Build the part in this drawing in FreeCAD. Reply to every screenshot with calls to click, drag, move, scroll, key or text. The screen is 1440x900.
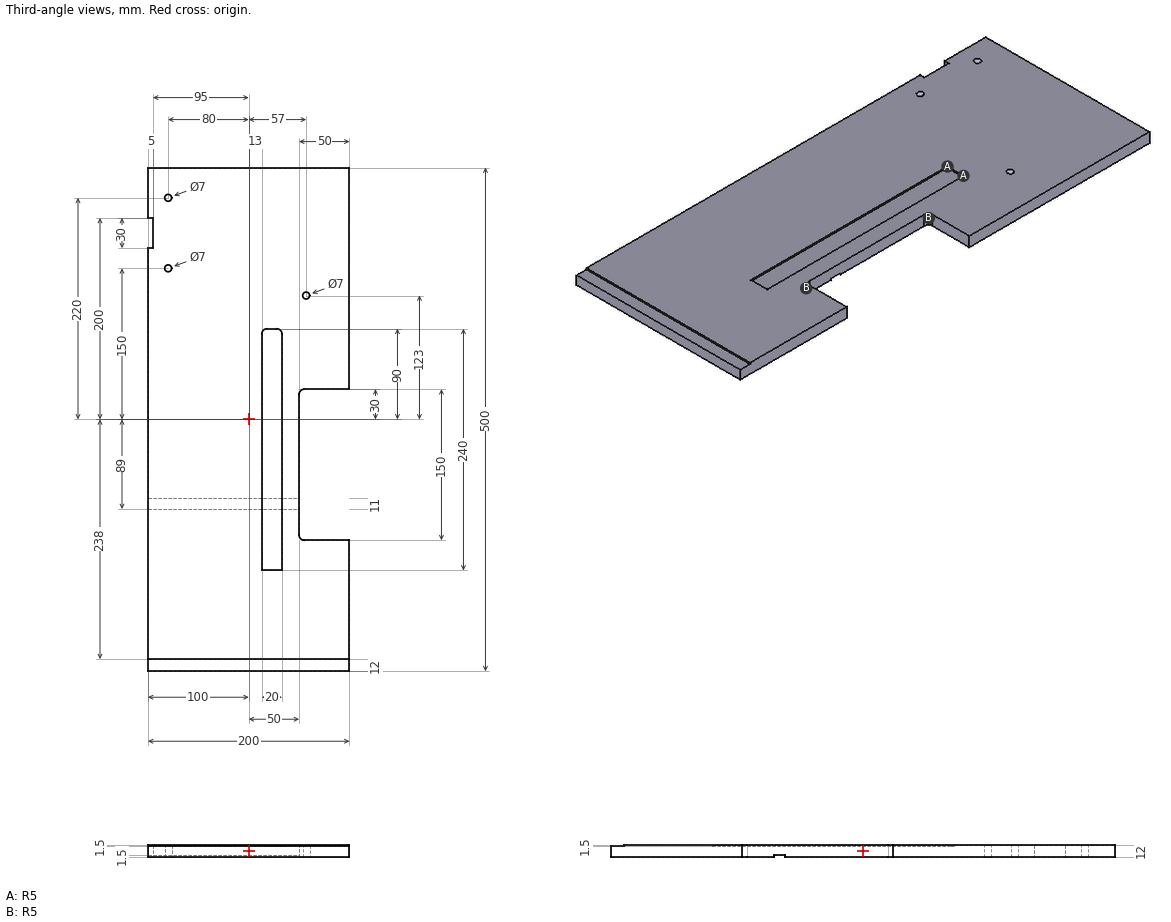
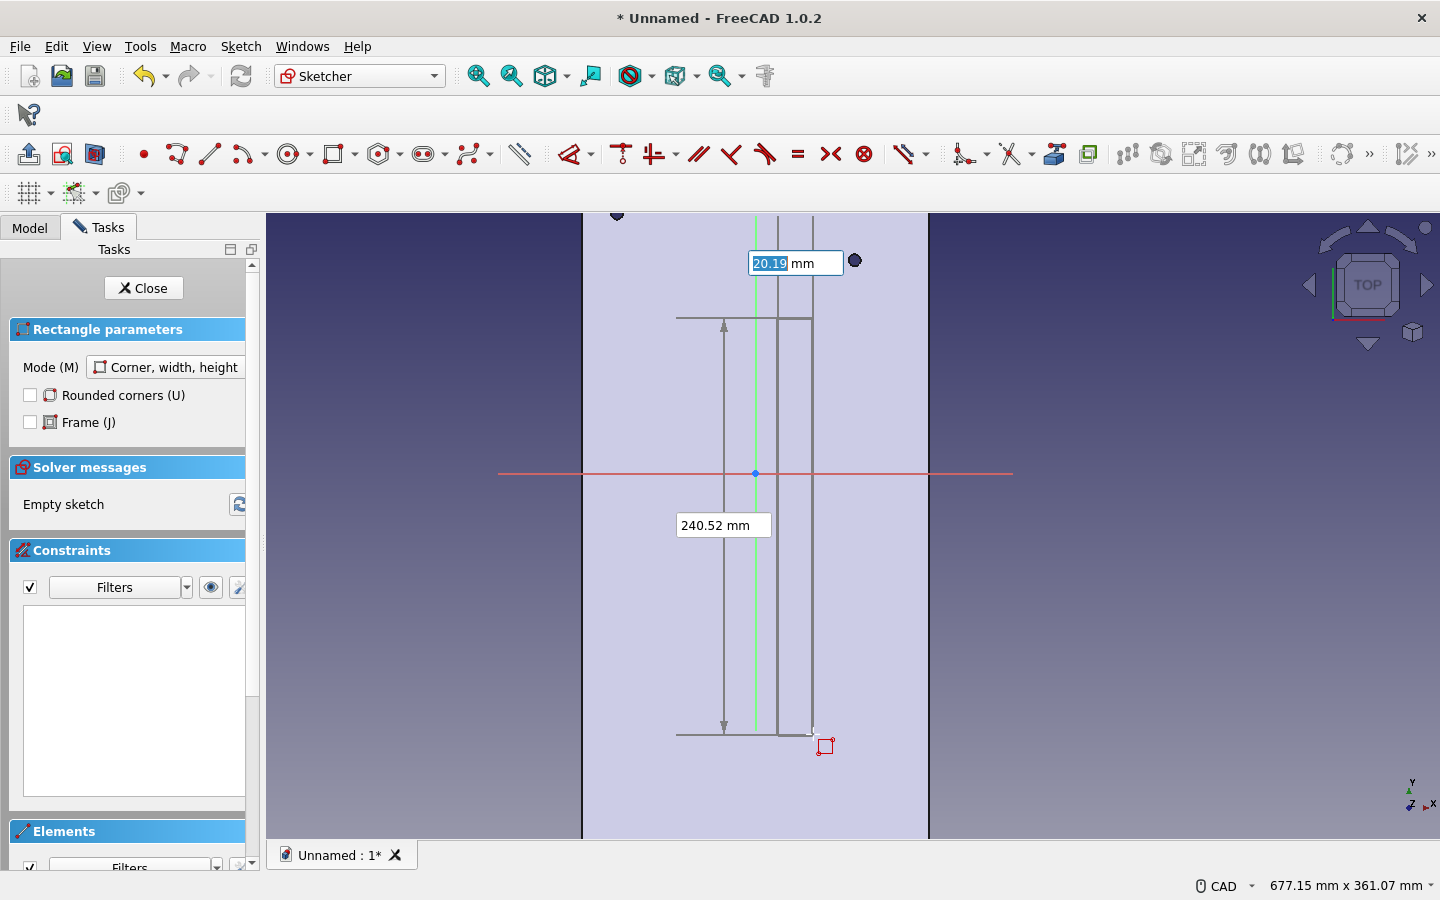
text(20)
key(Tab)
text(240)
key(Return)
key(Escape)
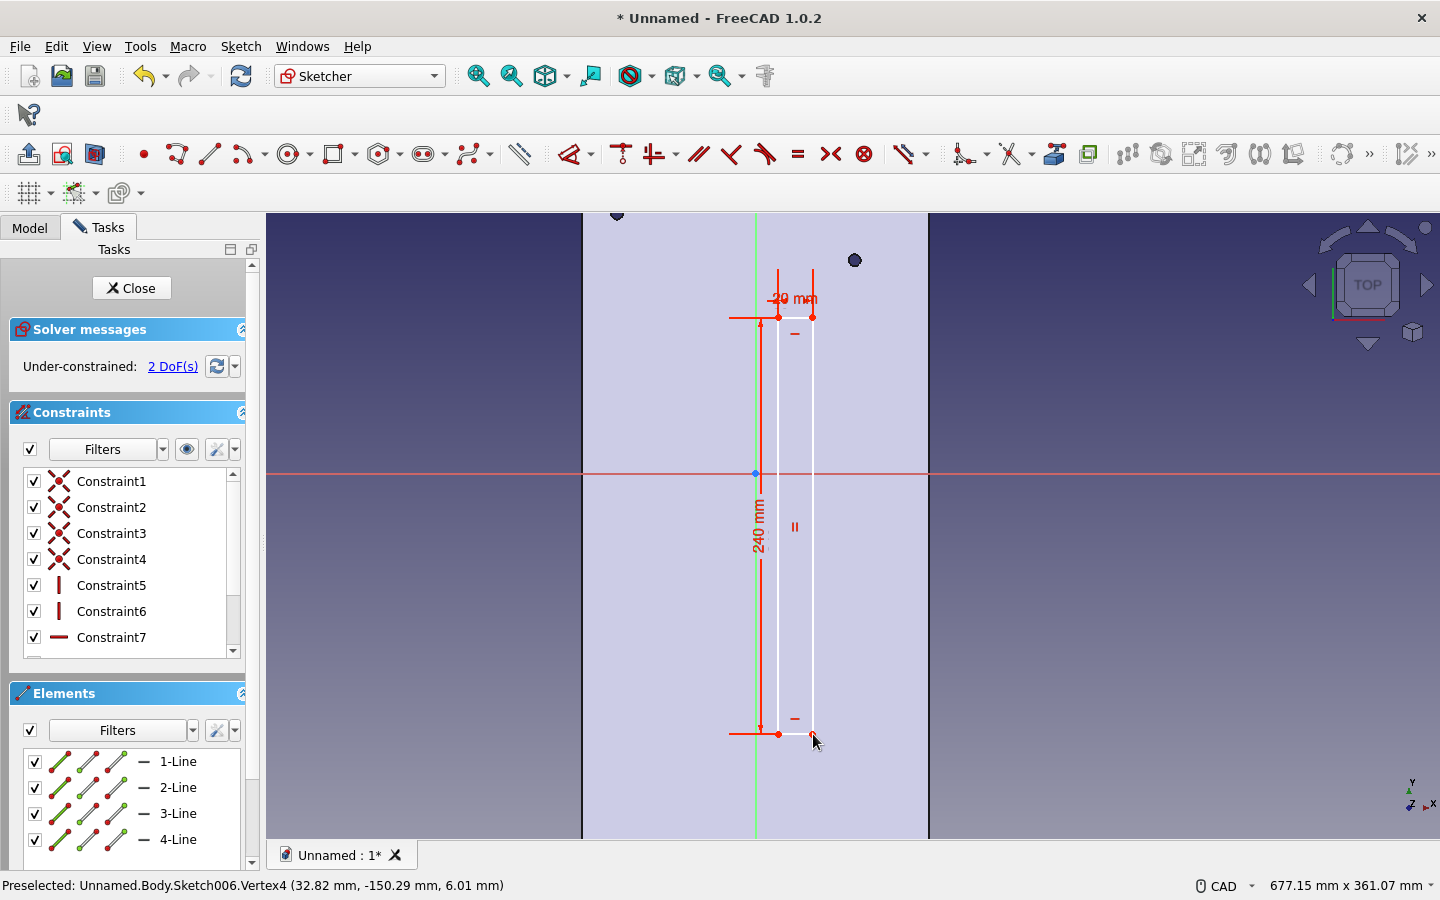
click(568, 154)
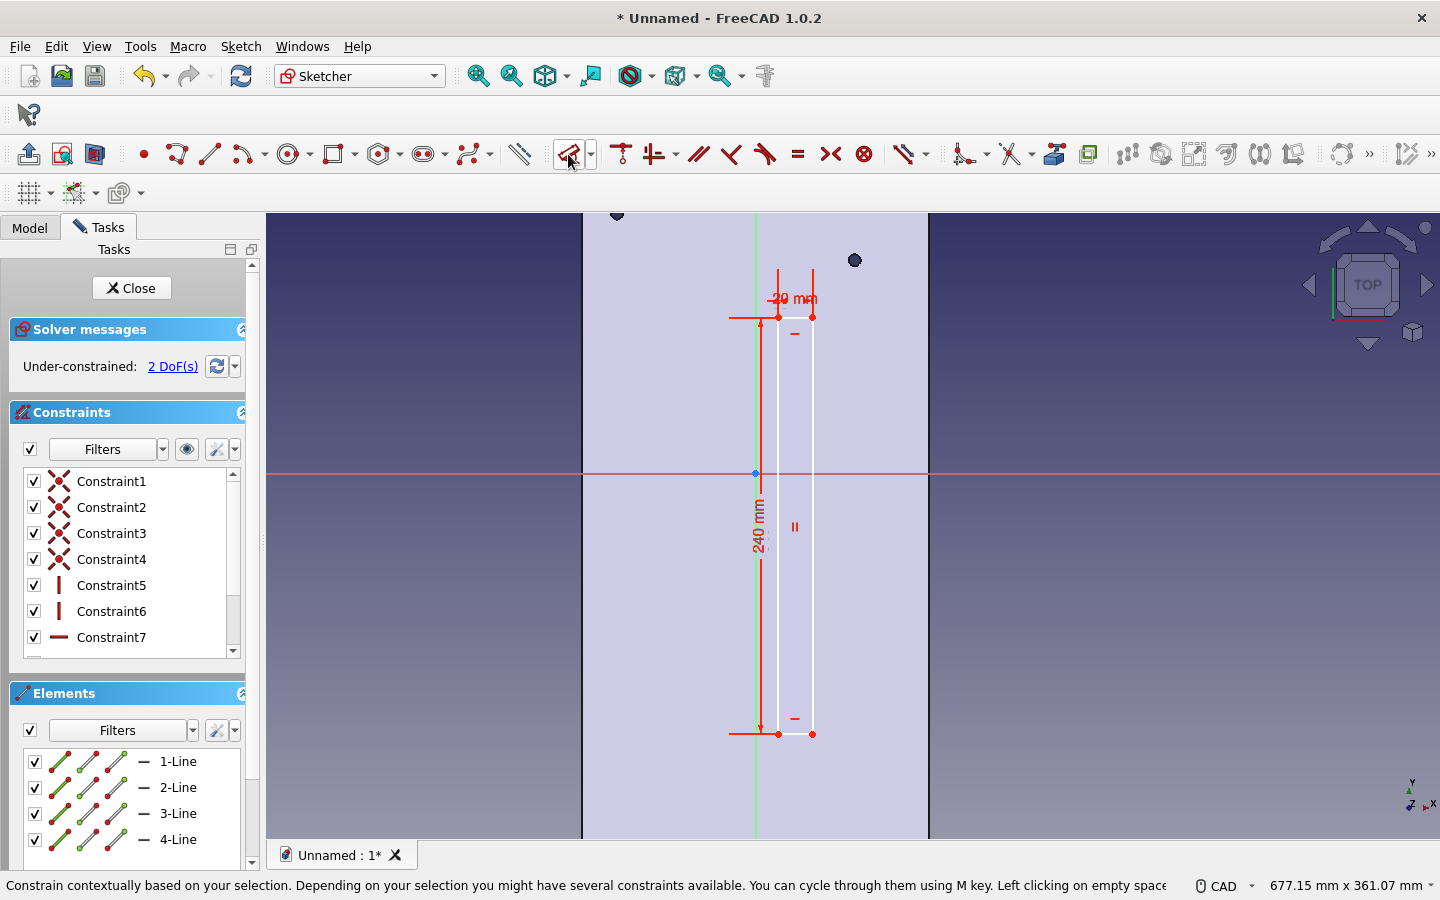
scroll(778, 318, up, 3)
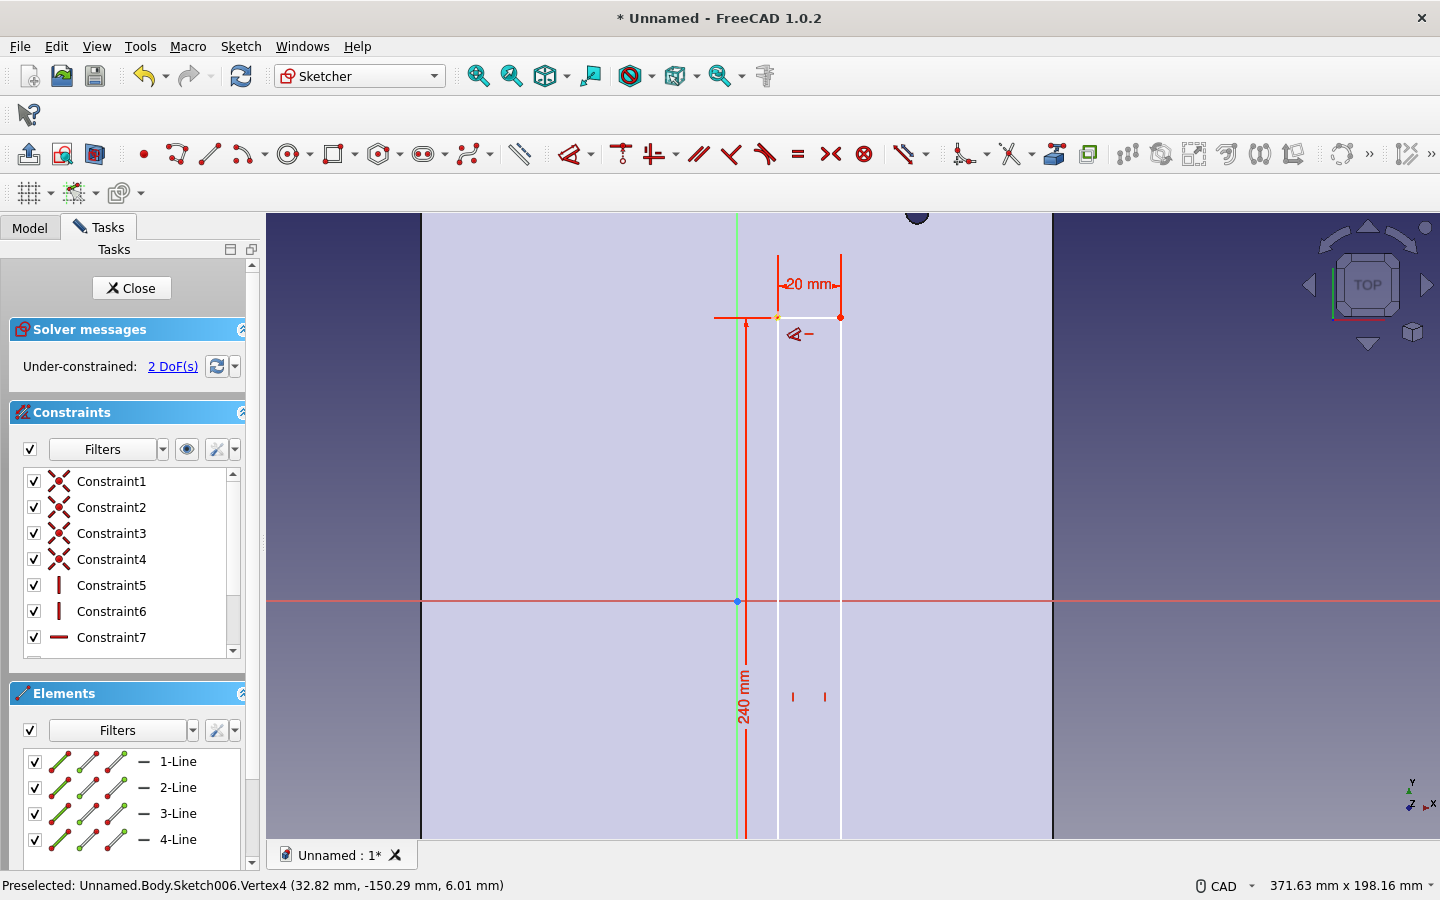
click(778, 318)
click(757, 284)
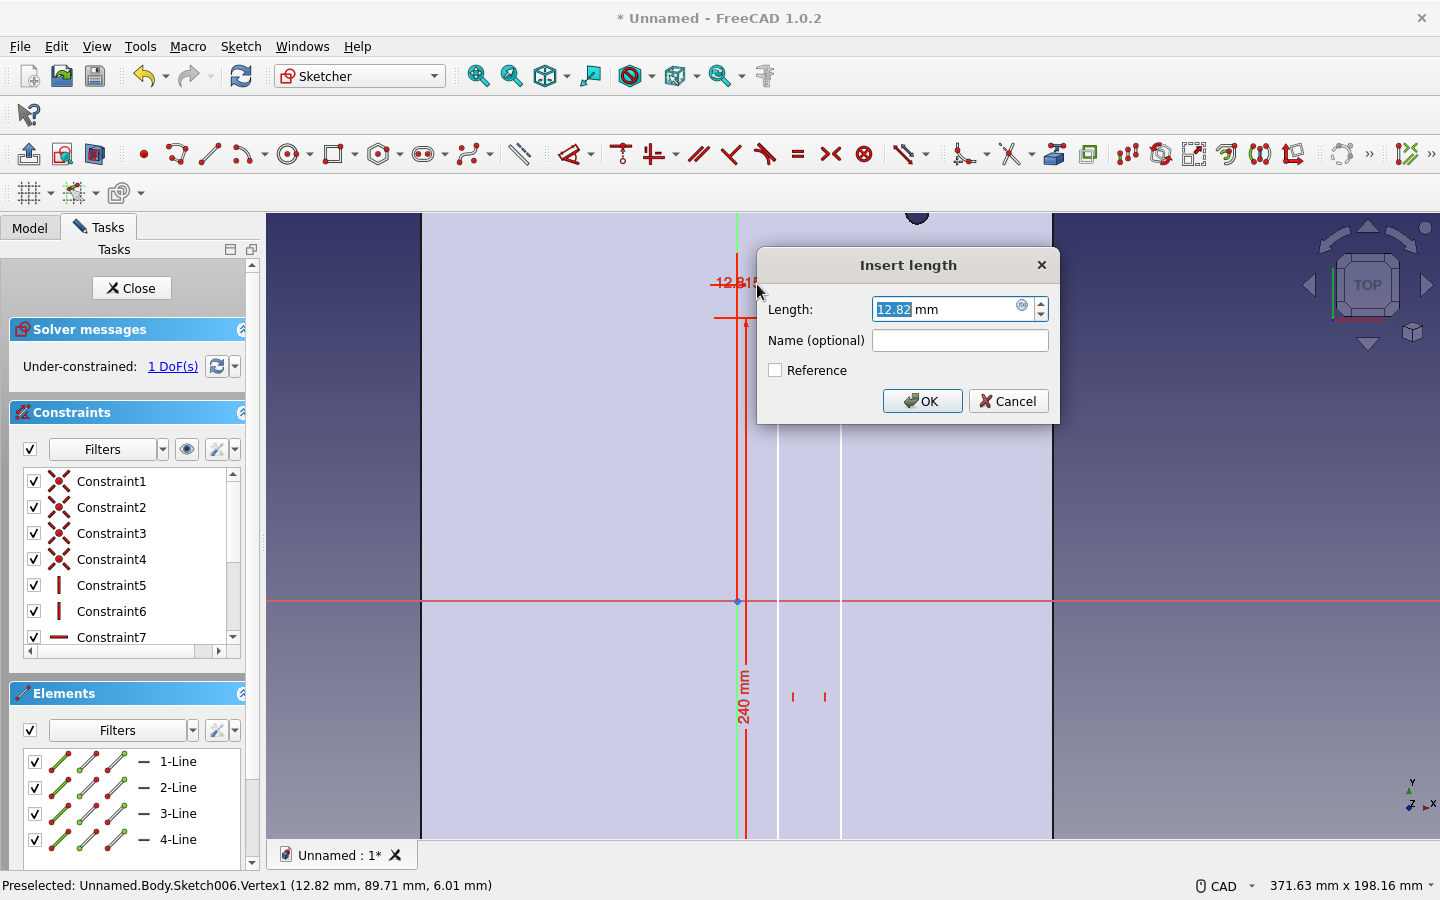
text(13)
key(Return)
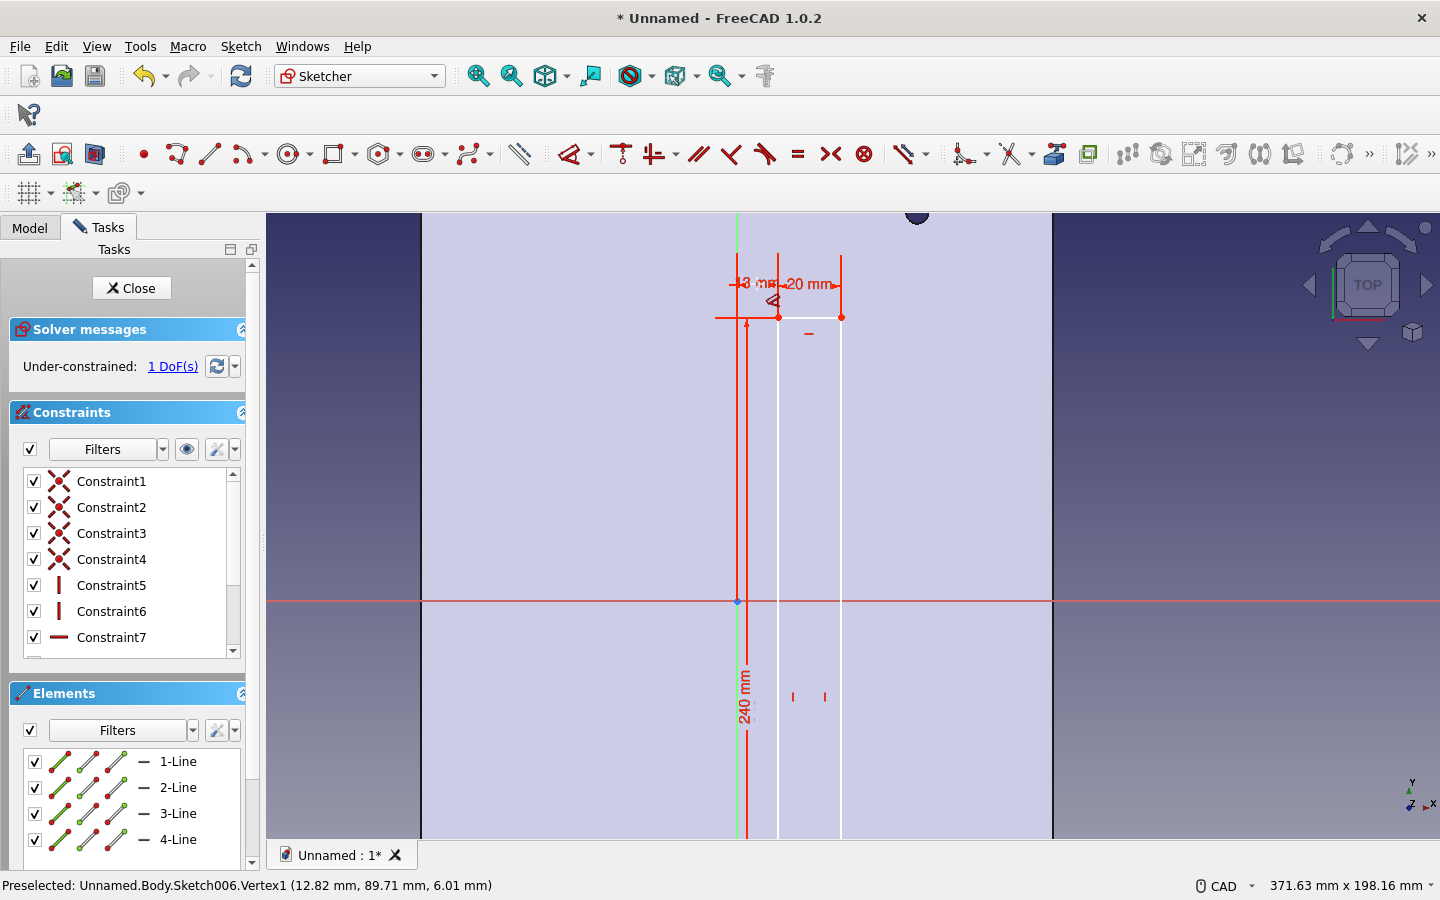
click(778, 318)
click(703, 460)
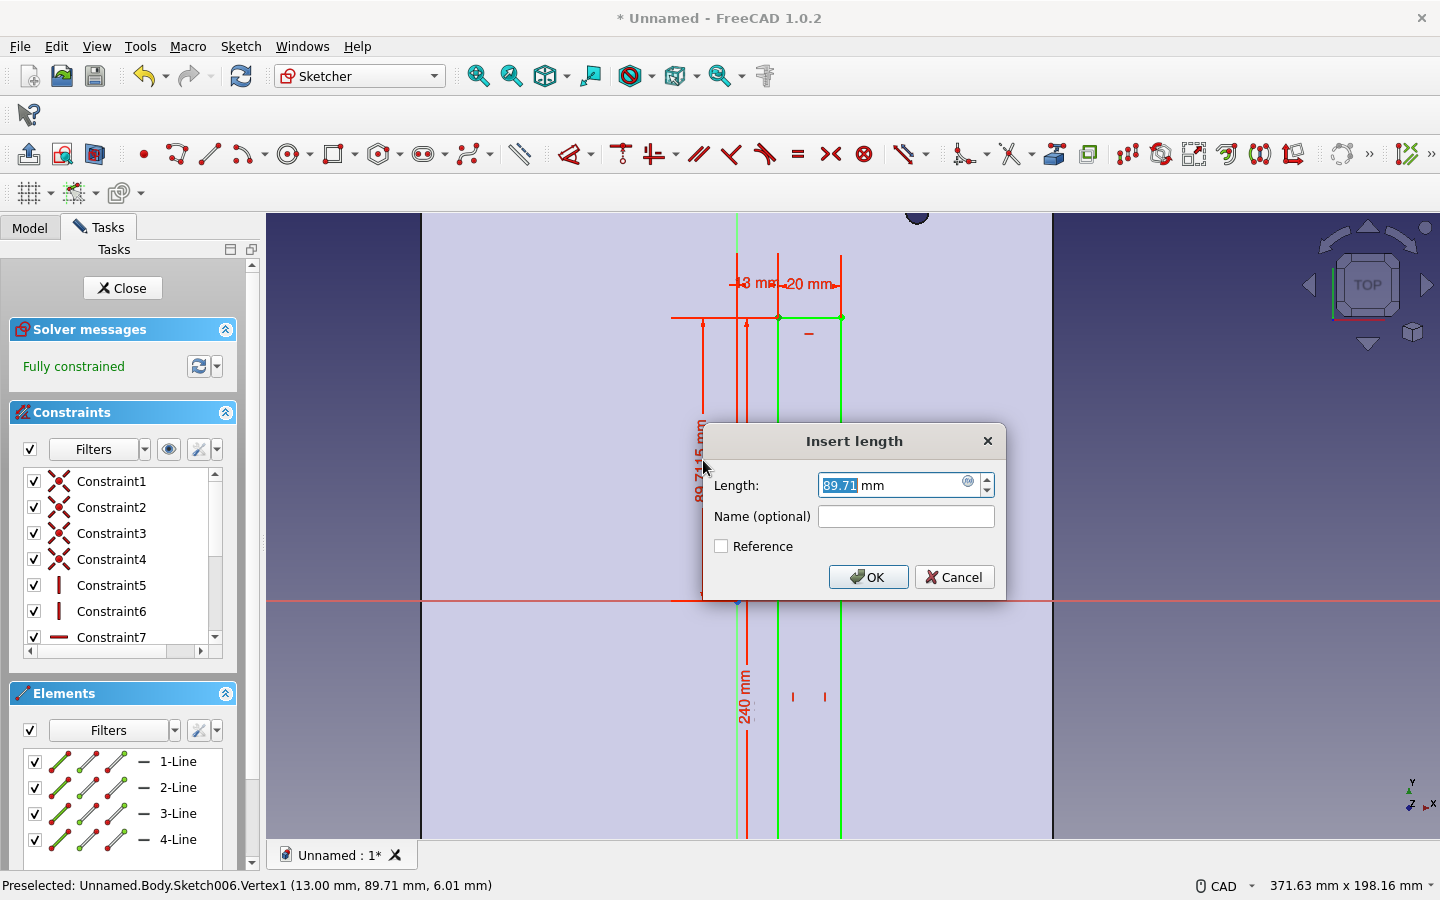
text(90)
key(Return)
key(Escape)